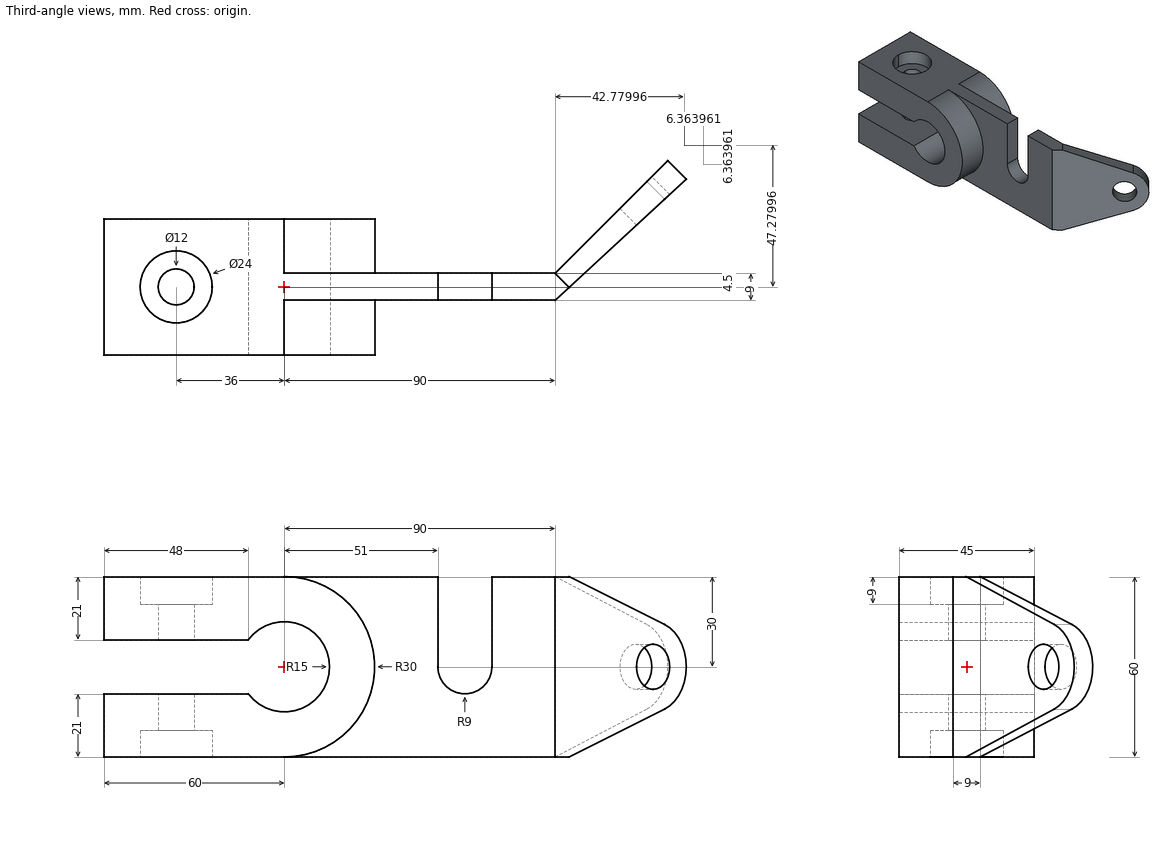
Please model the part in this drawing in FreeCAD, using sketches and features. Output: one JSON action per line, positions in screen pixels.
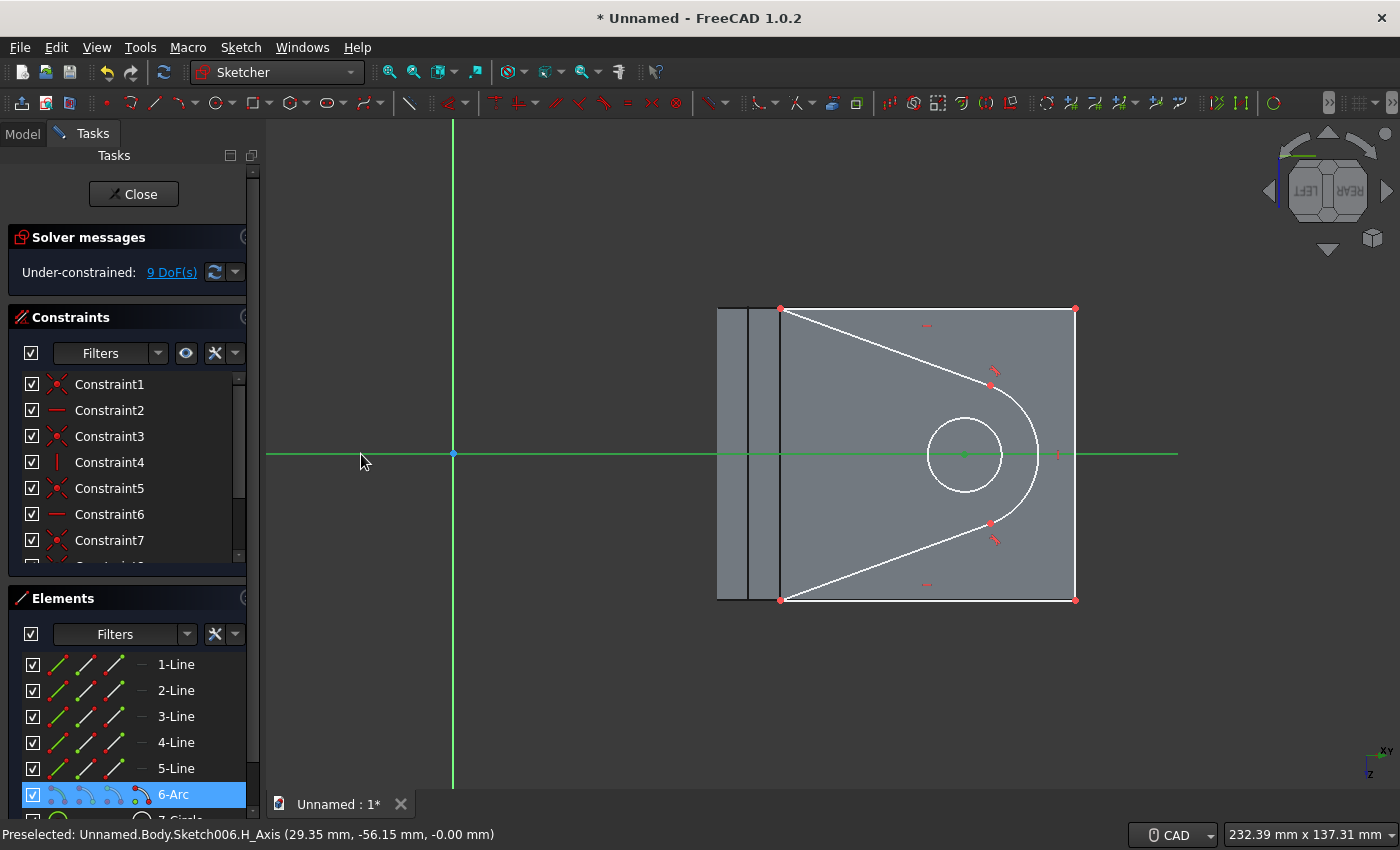
{"action": "left_click", "coordinate": [496, 104]}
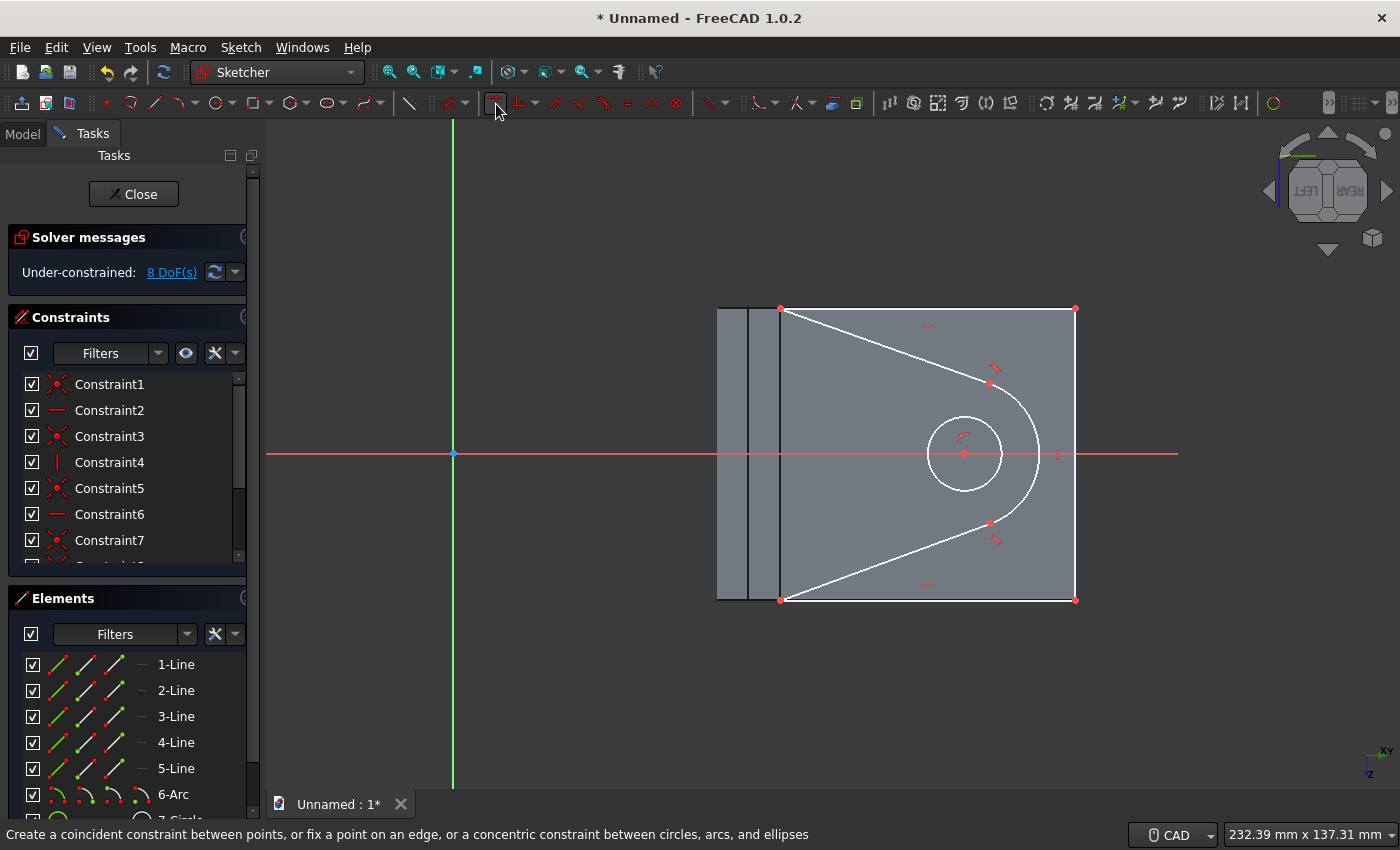
{"action": "key", "text": "d"}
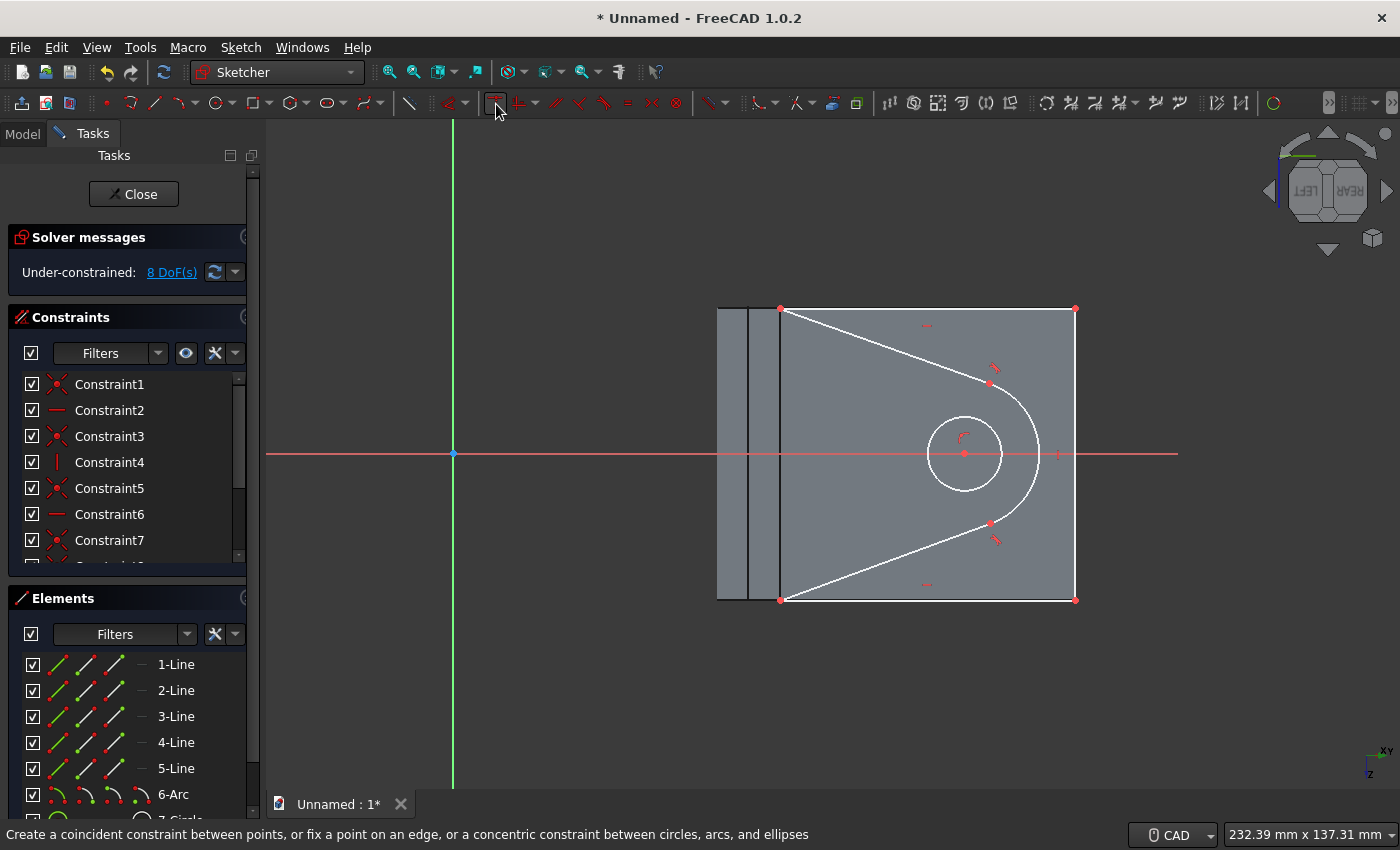
{"action": "left_click", "coordinate": [1031, 489]}
{"action": "left_click", "coordinate": [1059, 504]}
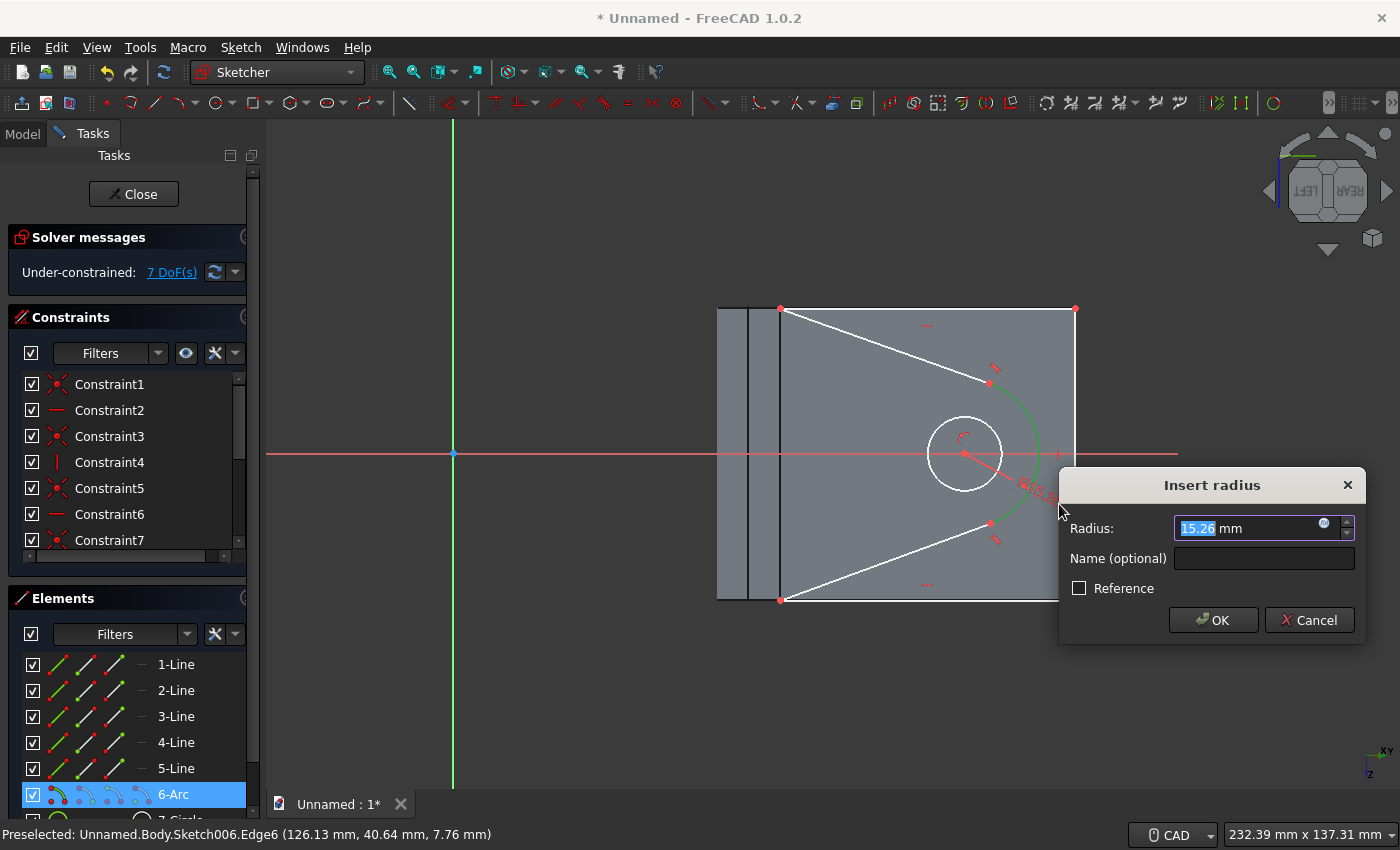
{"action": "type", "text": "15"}
{"action": "key", "text": "Return"}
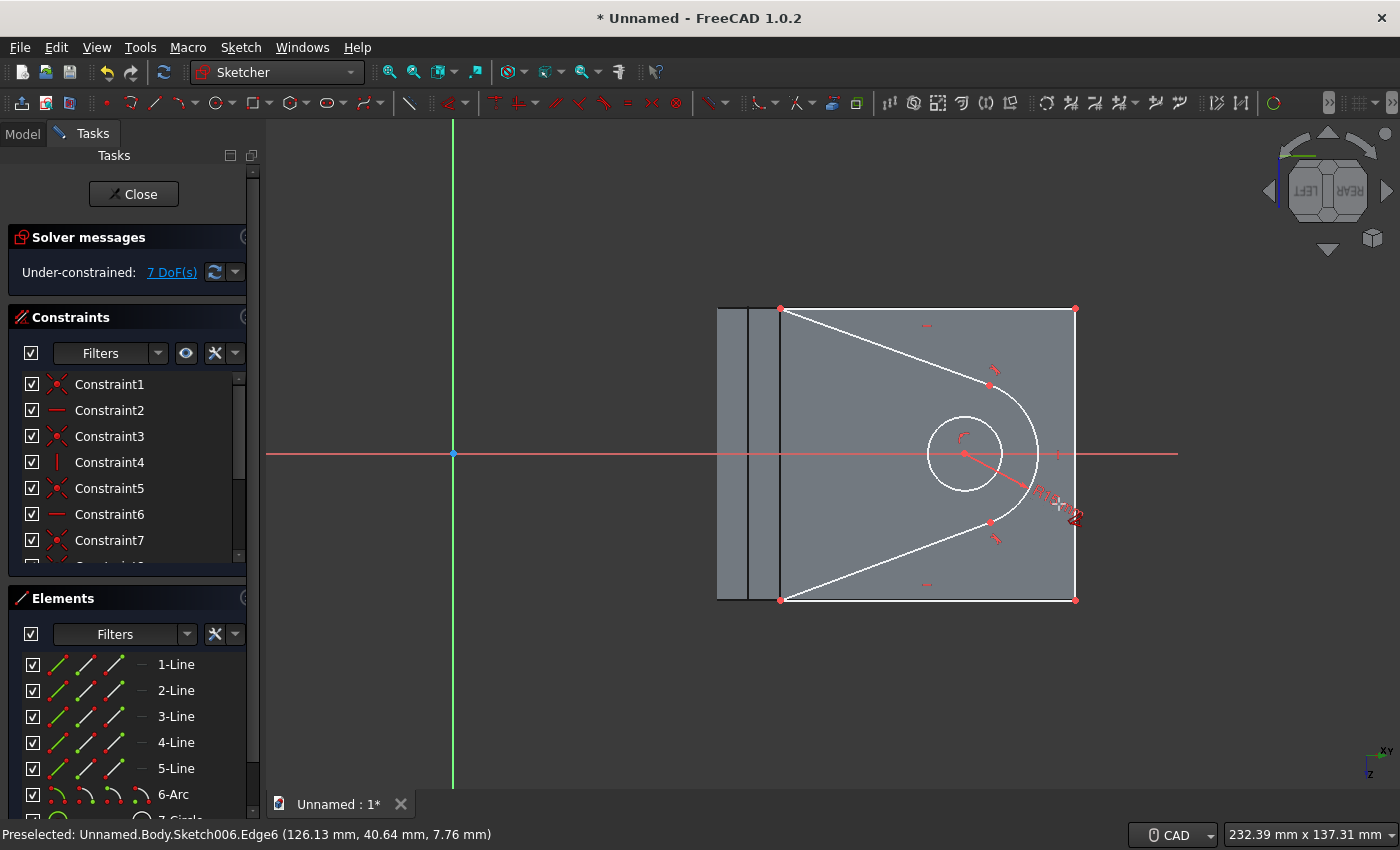
{"action": "left_click", "coordinate": [991, 428]}
{"action": "left_click", "coordinate": [951, 387]}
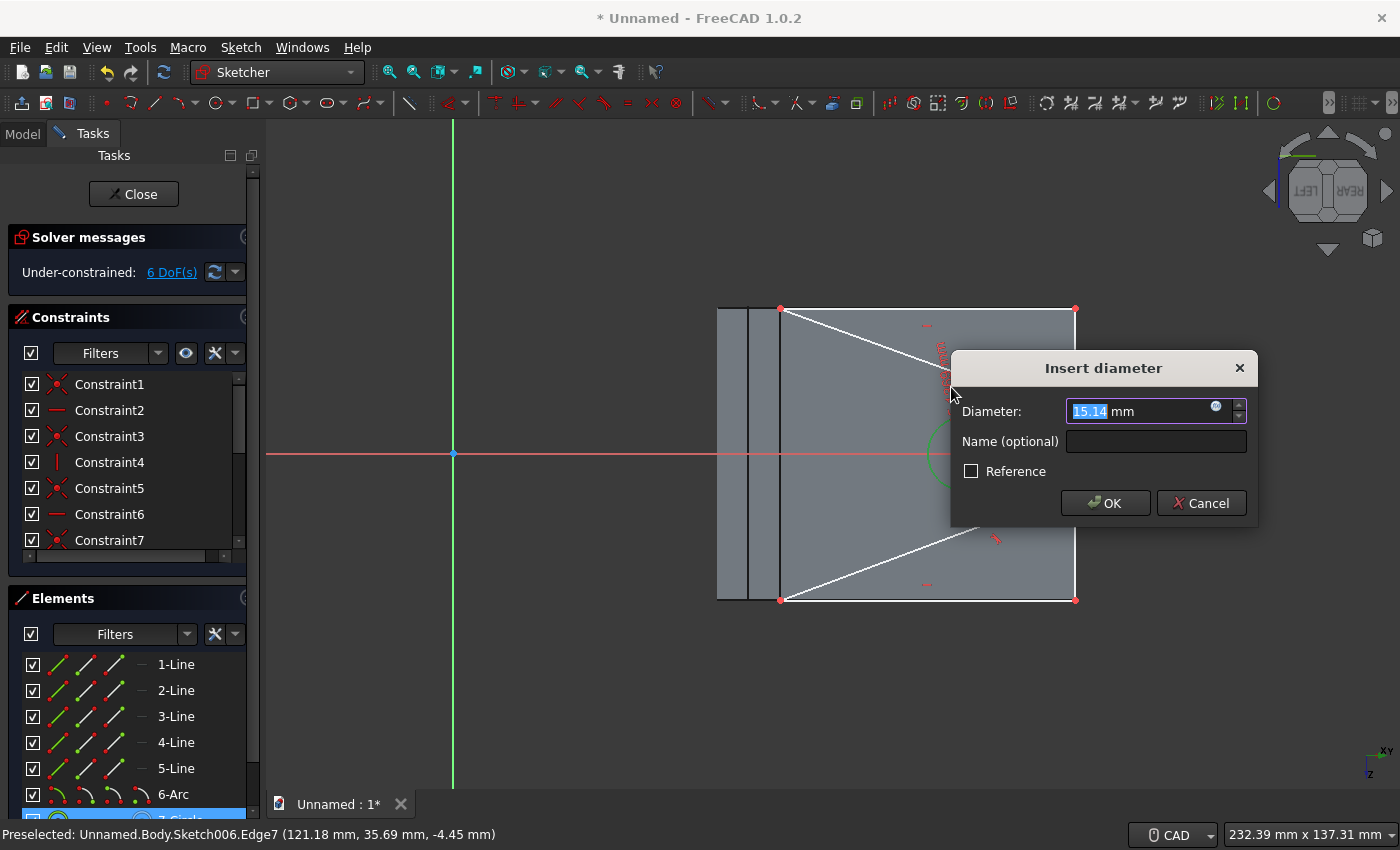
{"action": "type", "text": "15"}
{"action": "key", "text": "Return"}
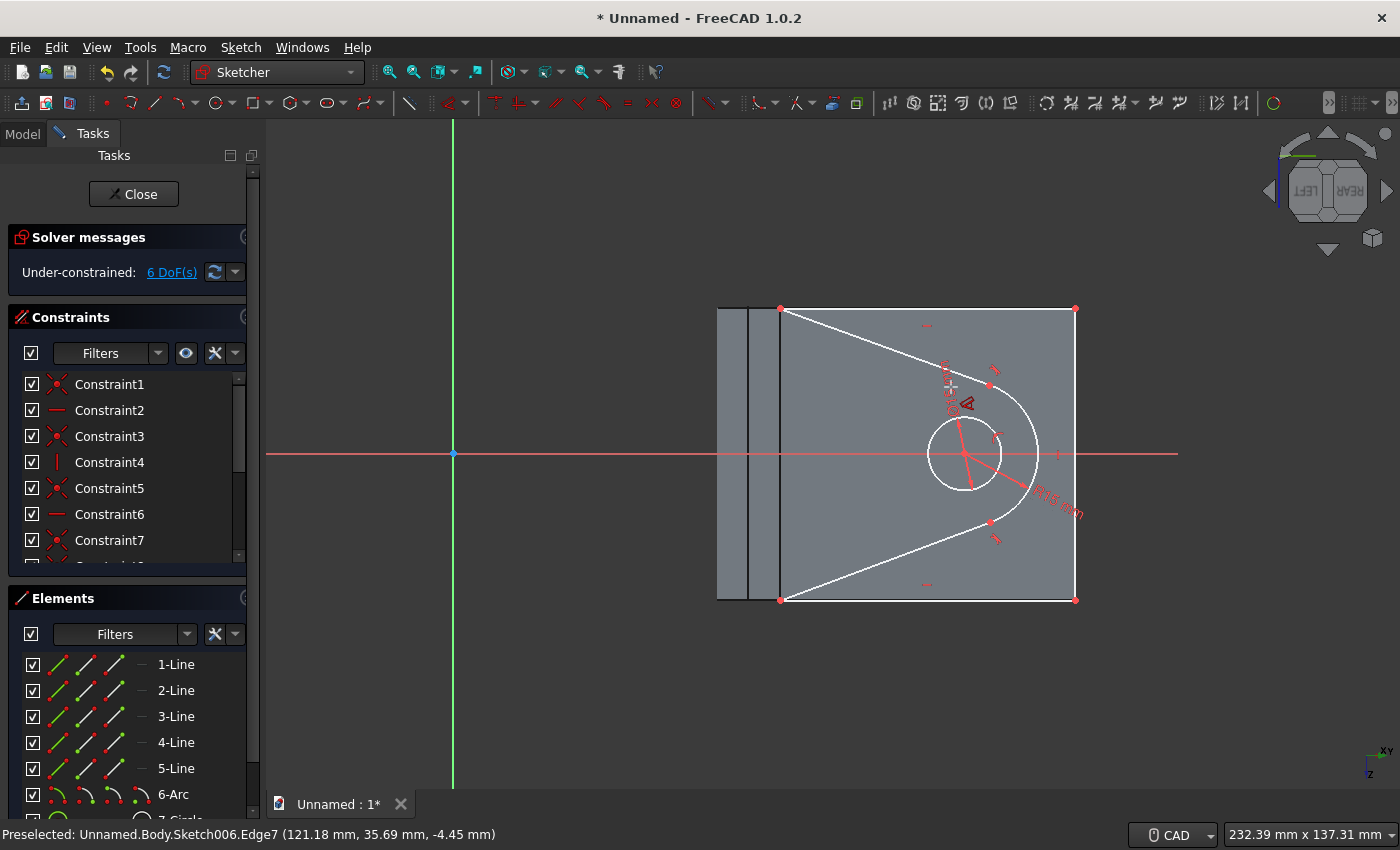
{"action": "left_click", "coordinate": [1075, 513]}
{"action": "left_click", "coordinate": [1109, 388]}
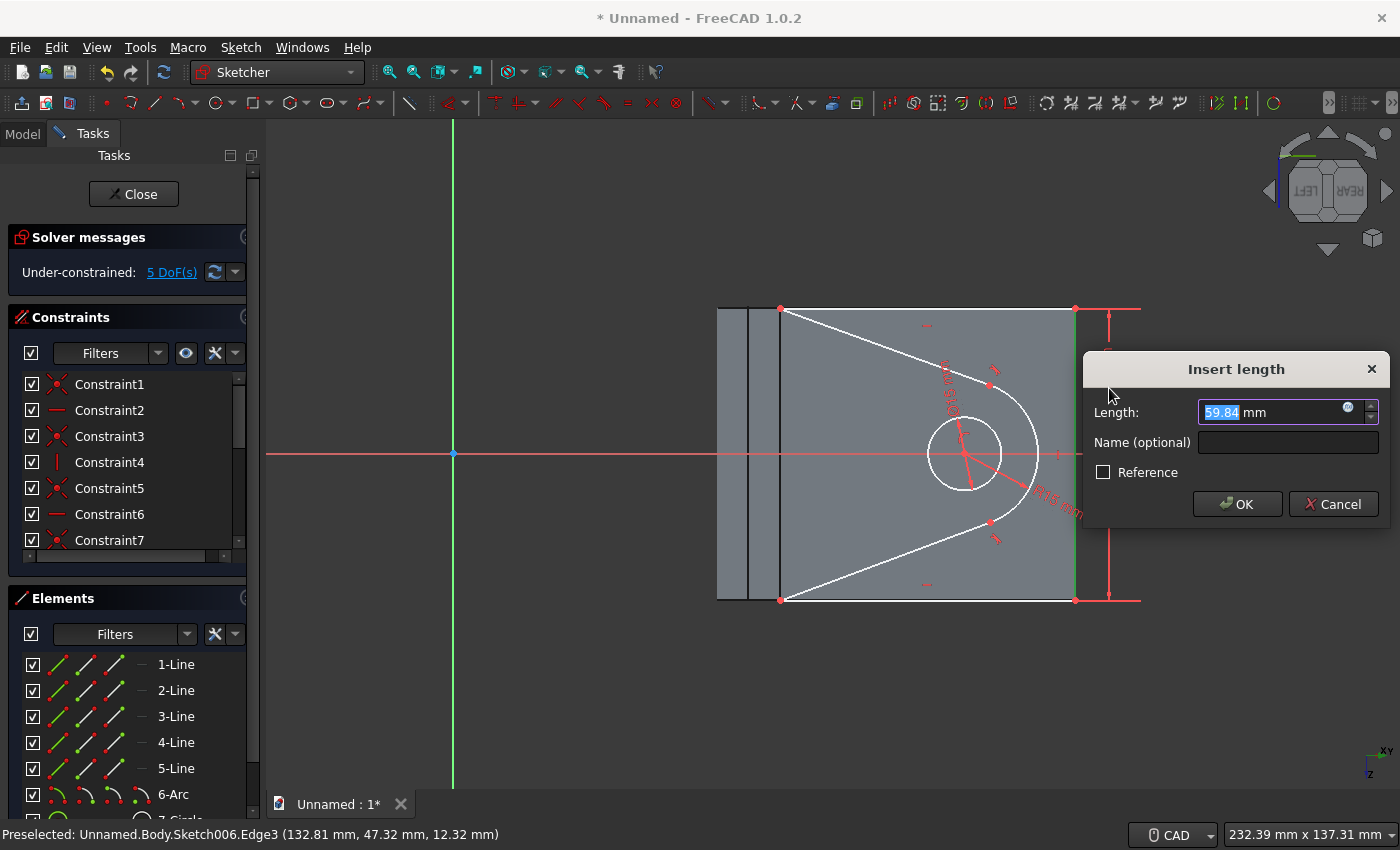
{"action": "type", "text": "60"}
{"action": "key", "text": "Return"}